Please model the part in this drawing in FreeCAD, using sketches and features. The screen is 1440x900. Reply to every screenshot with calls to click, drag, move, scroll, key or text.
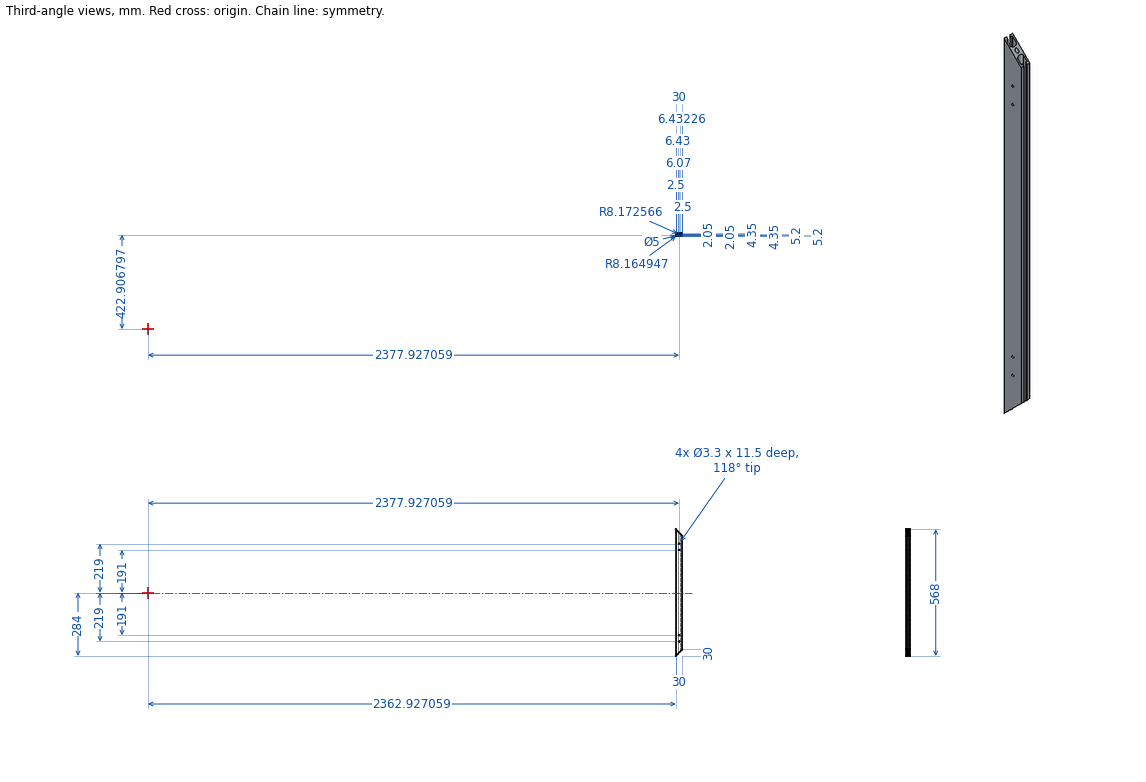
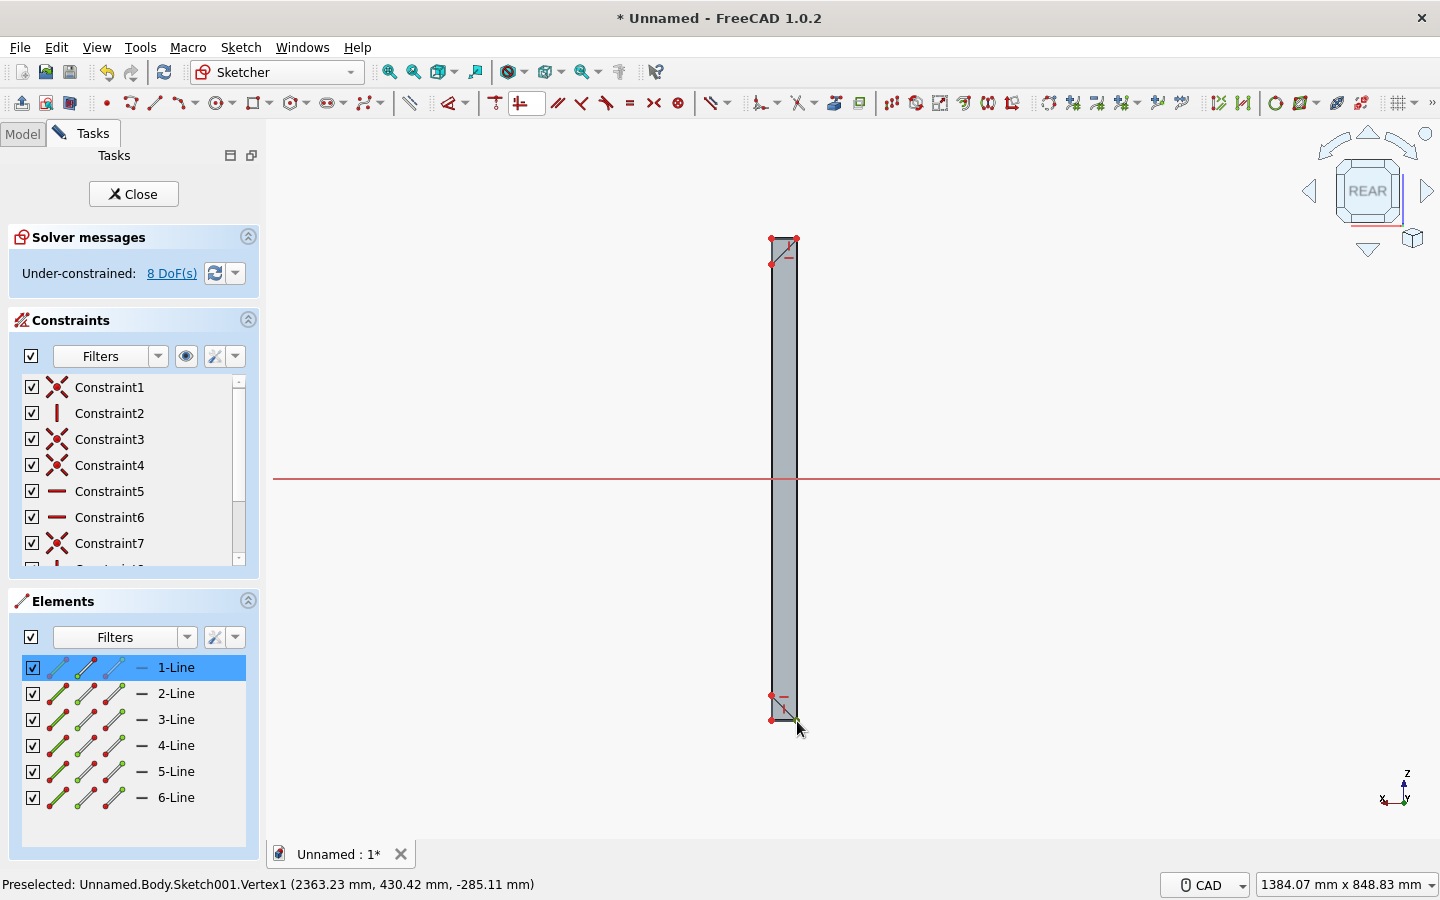
click(797, 239)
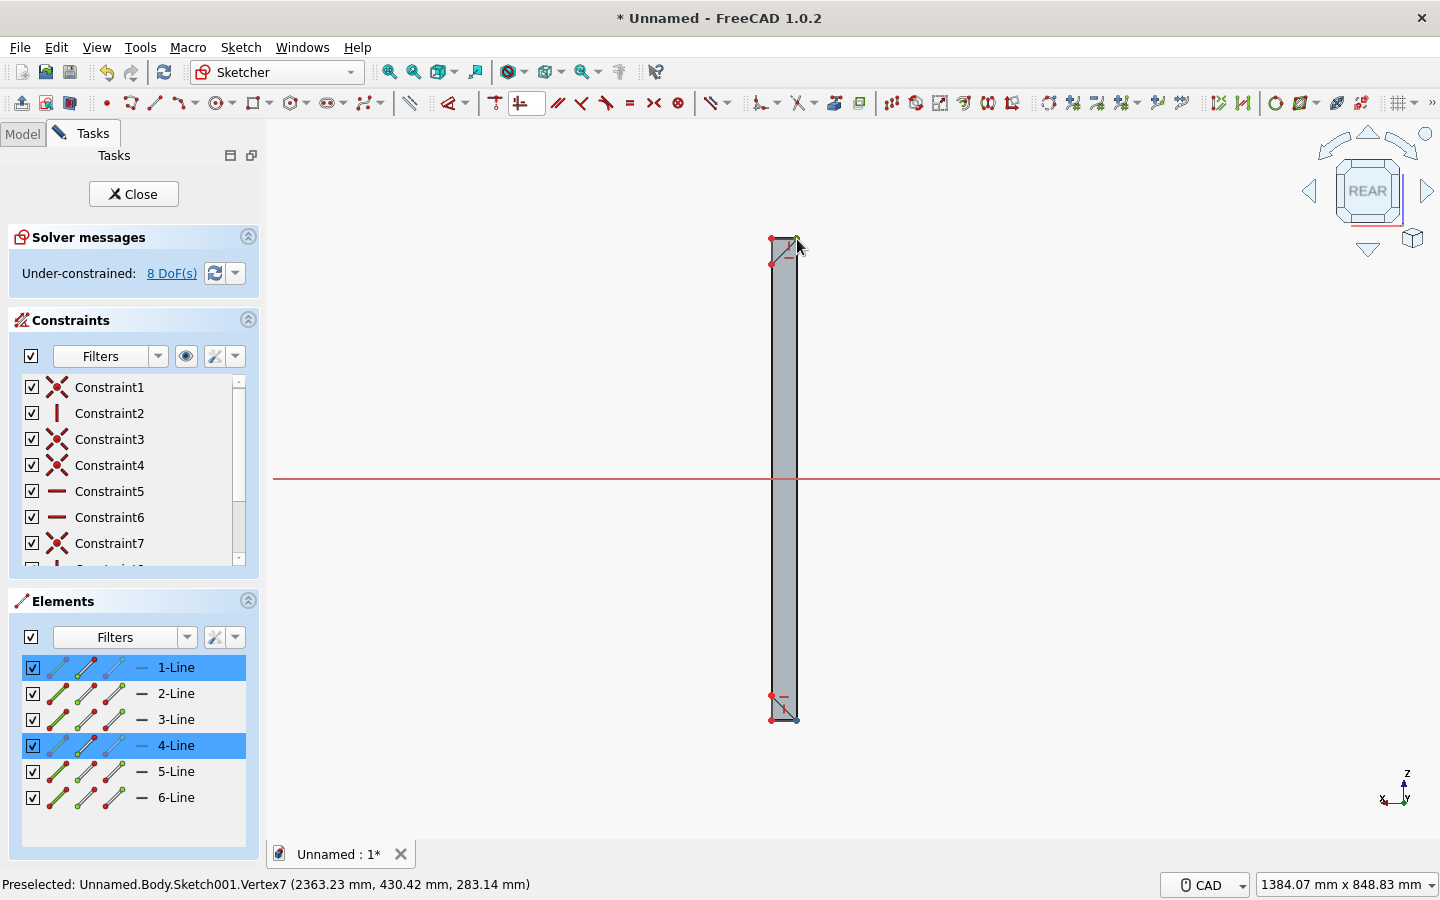
click(364, 479)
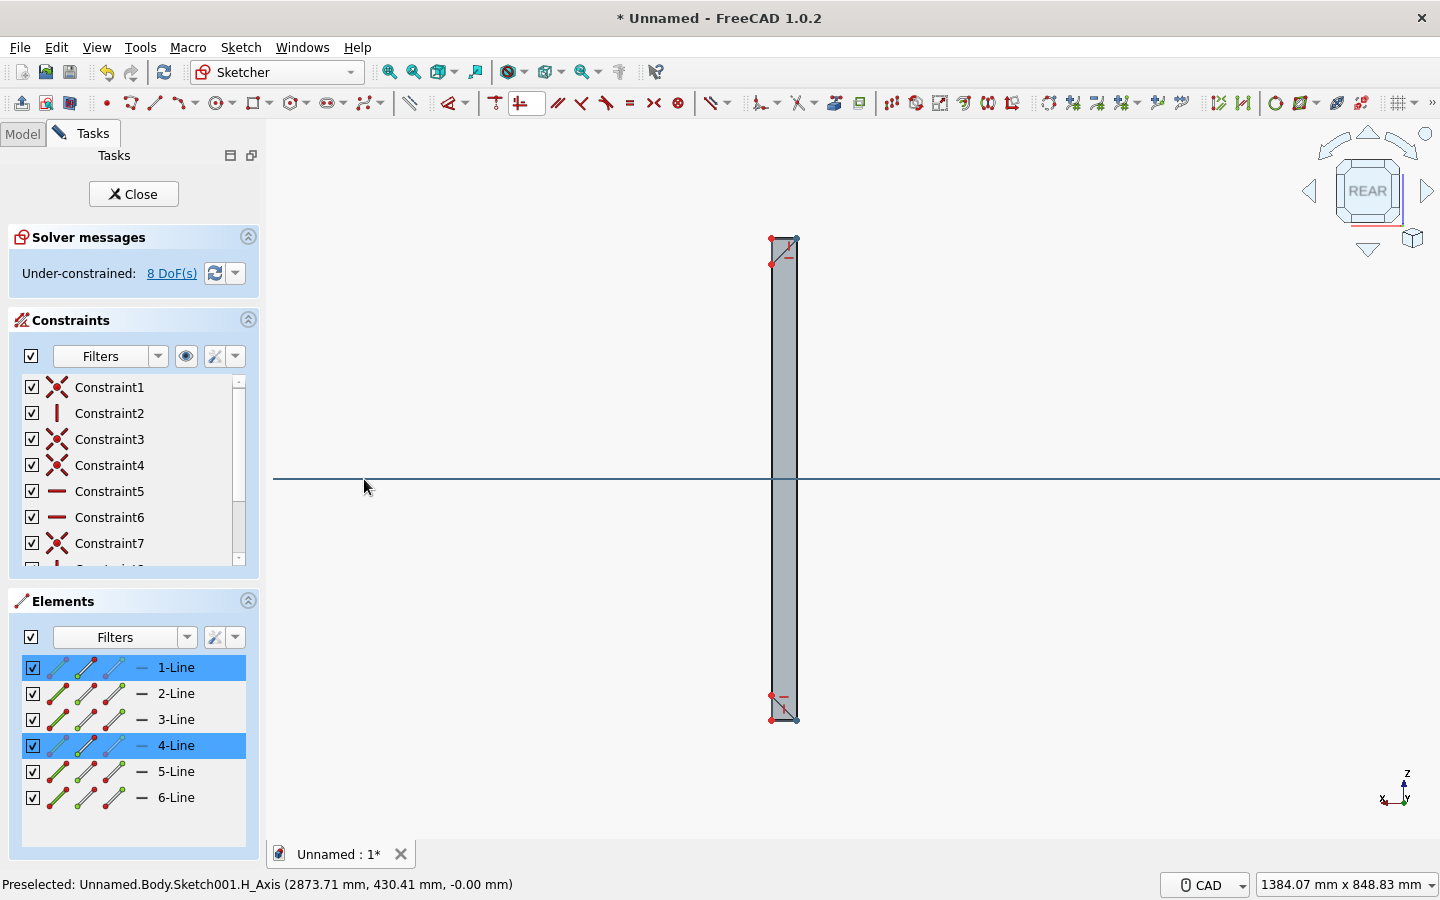
key(s)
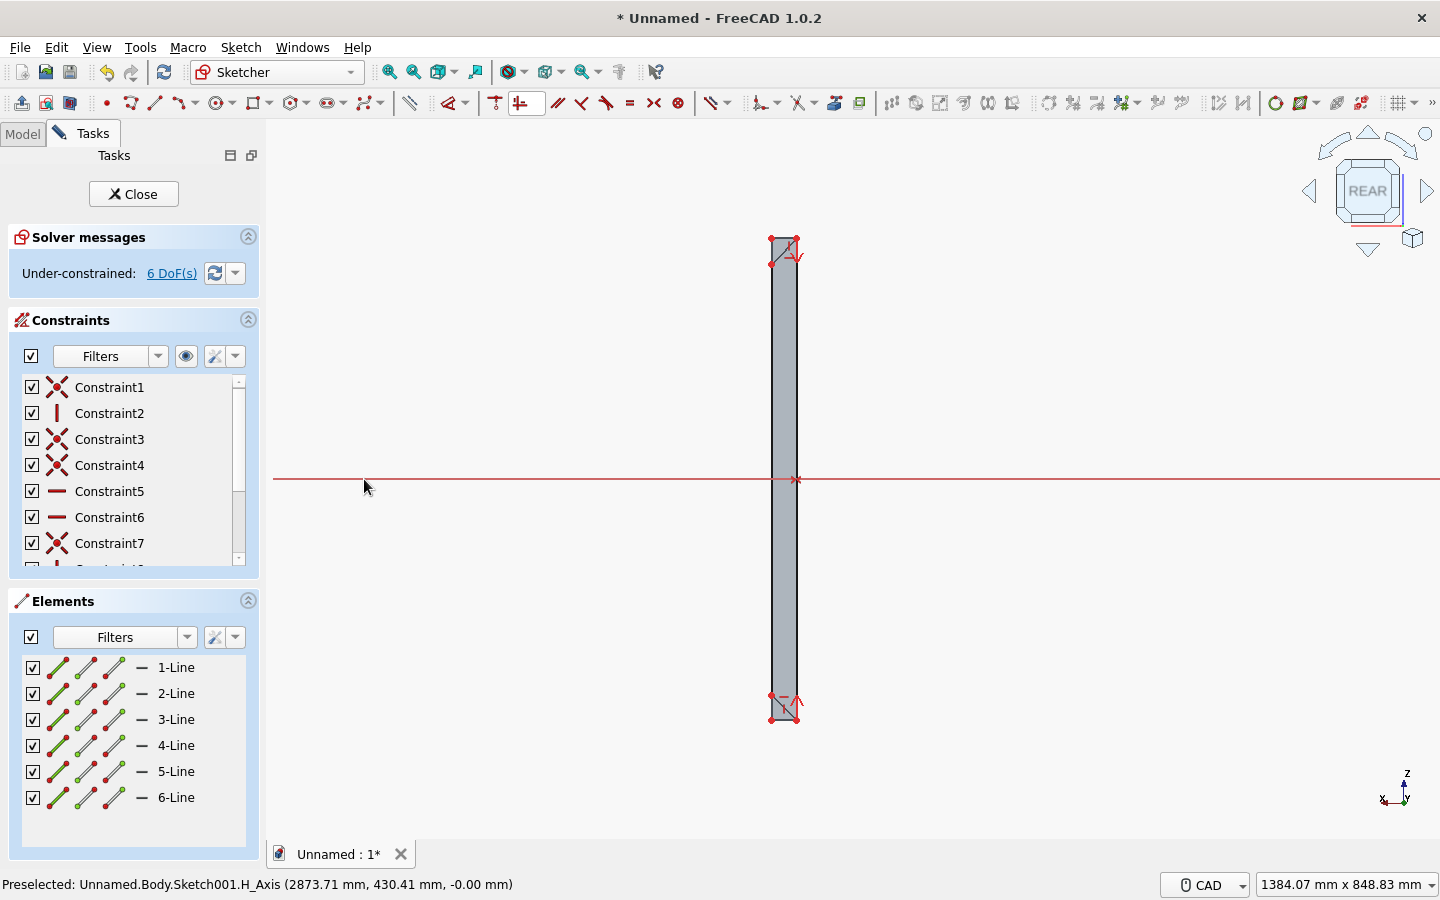
click(772, 696)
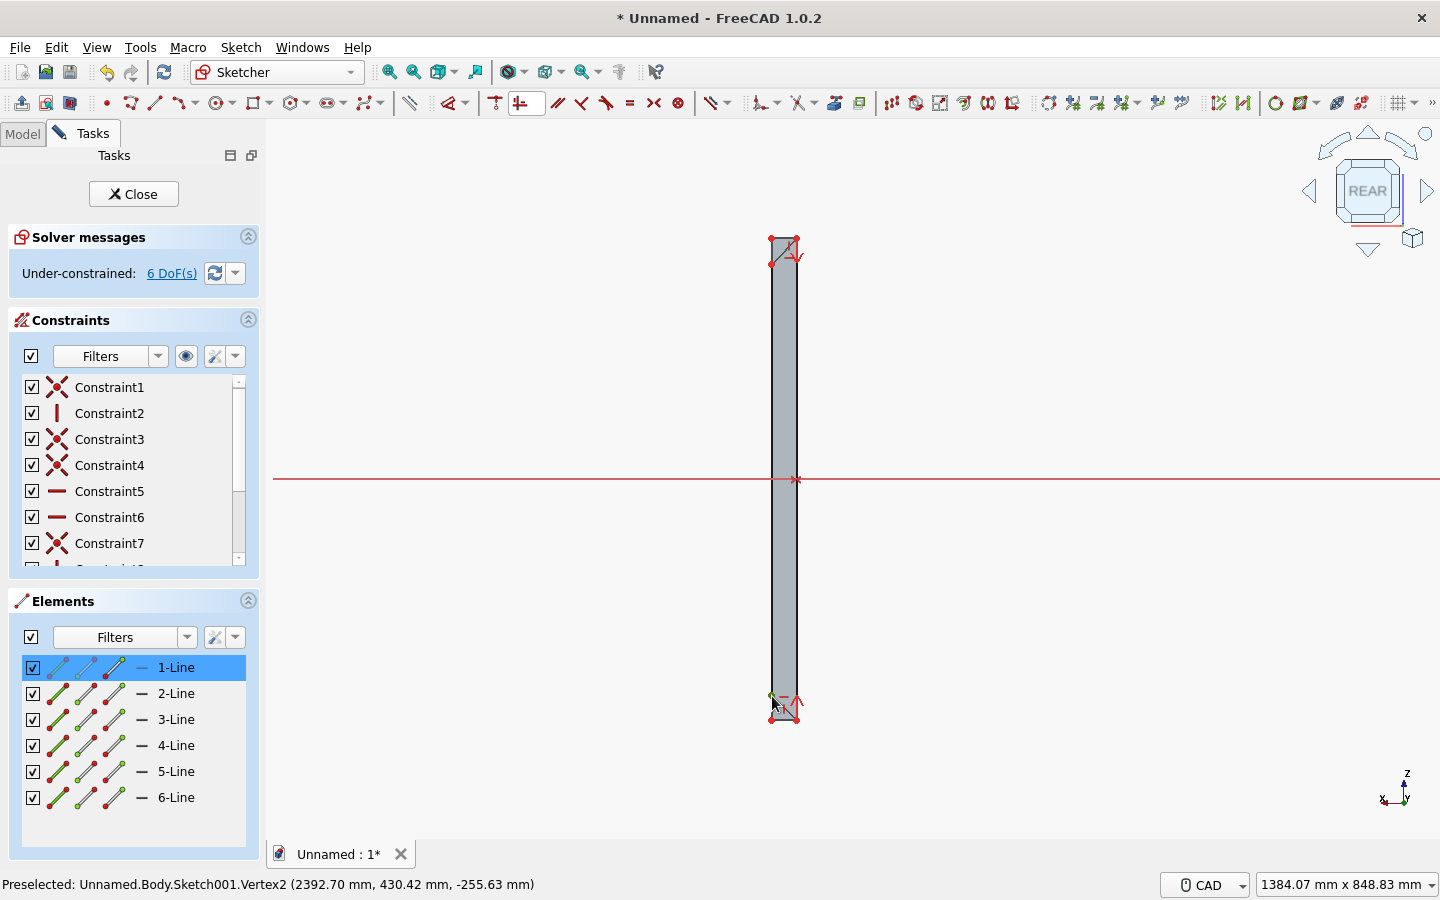
click(772, 265)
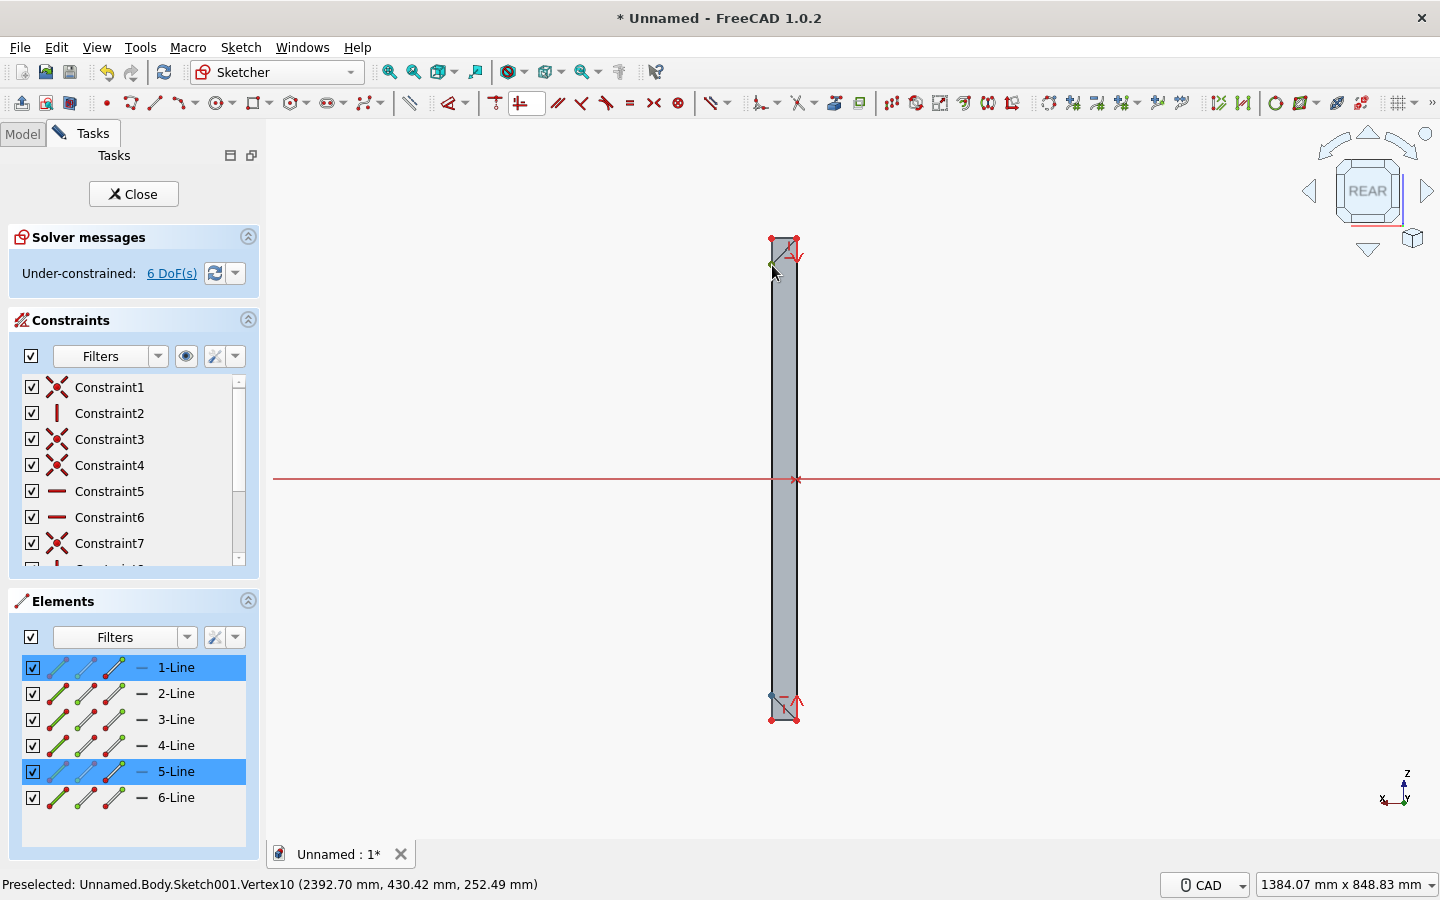
click(364, 479)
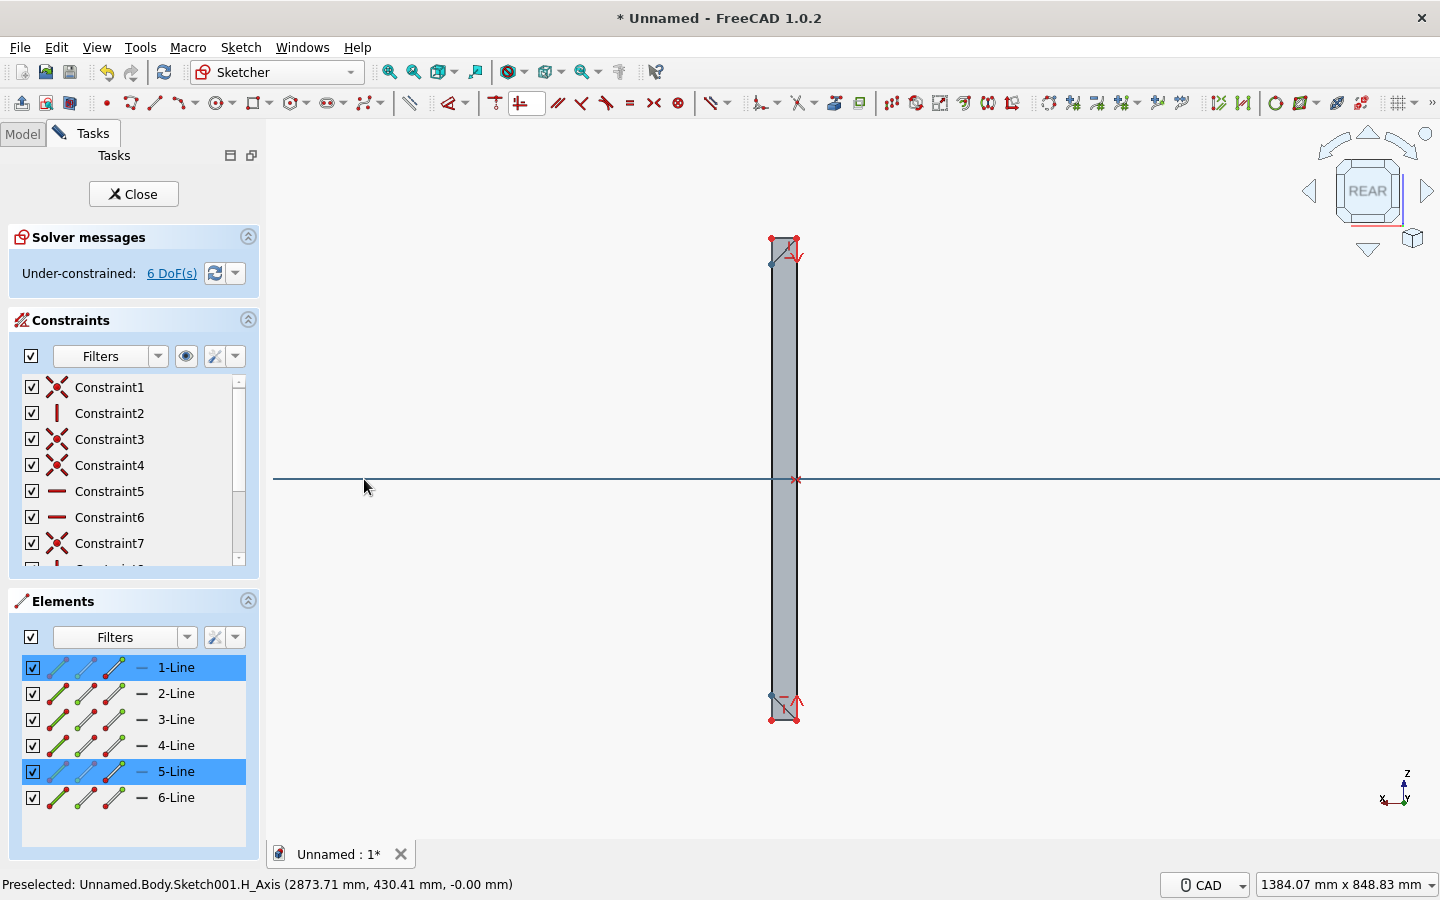
key(s)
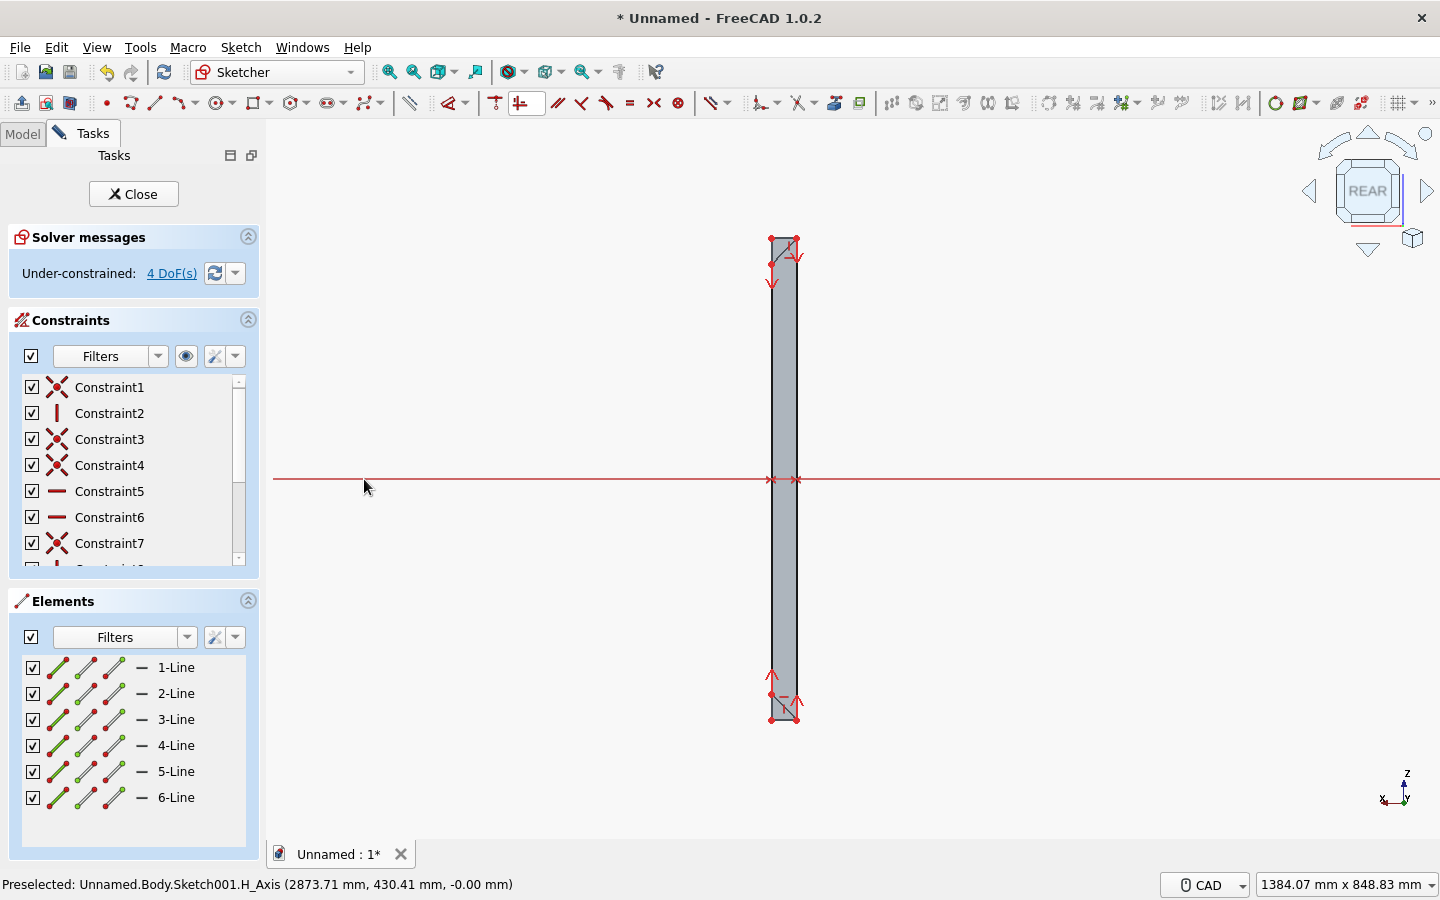
click(448, 104)